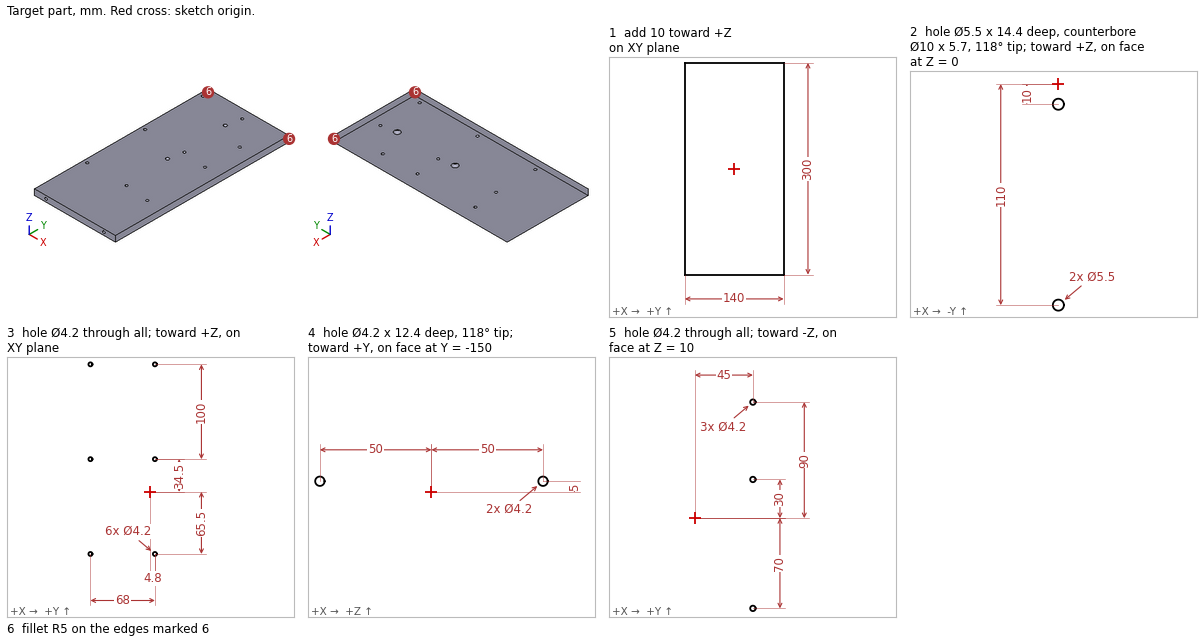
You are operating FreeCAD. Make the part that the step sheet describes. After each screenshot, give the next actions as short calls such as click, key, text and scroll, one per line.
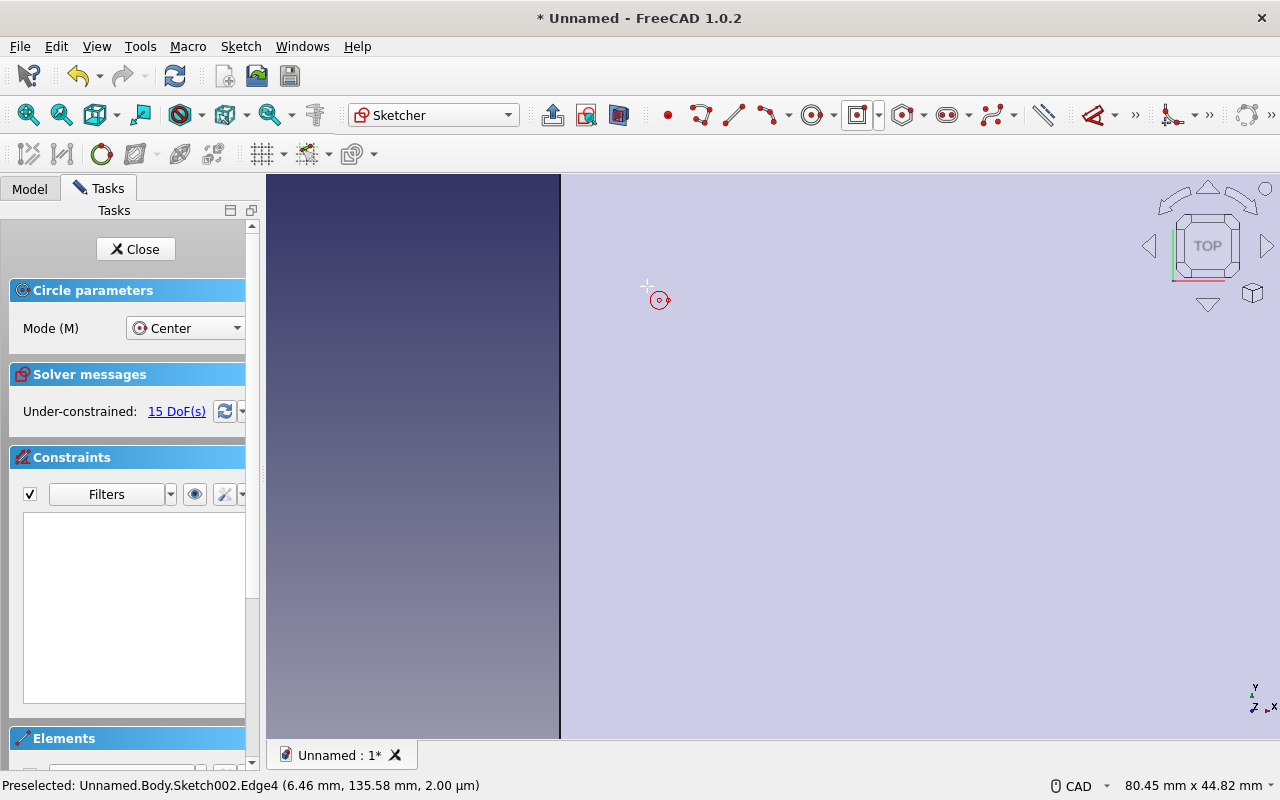
scroll(647, 286, down, 10)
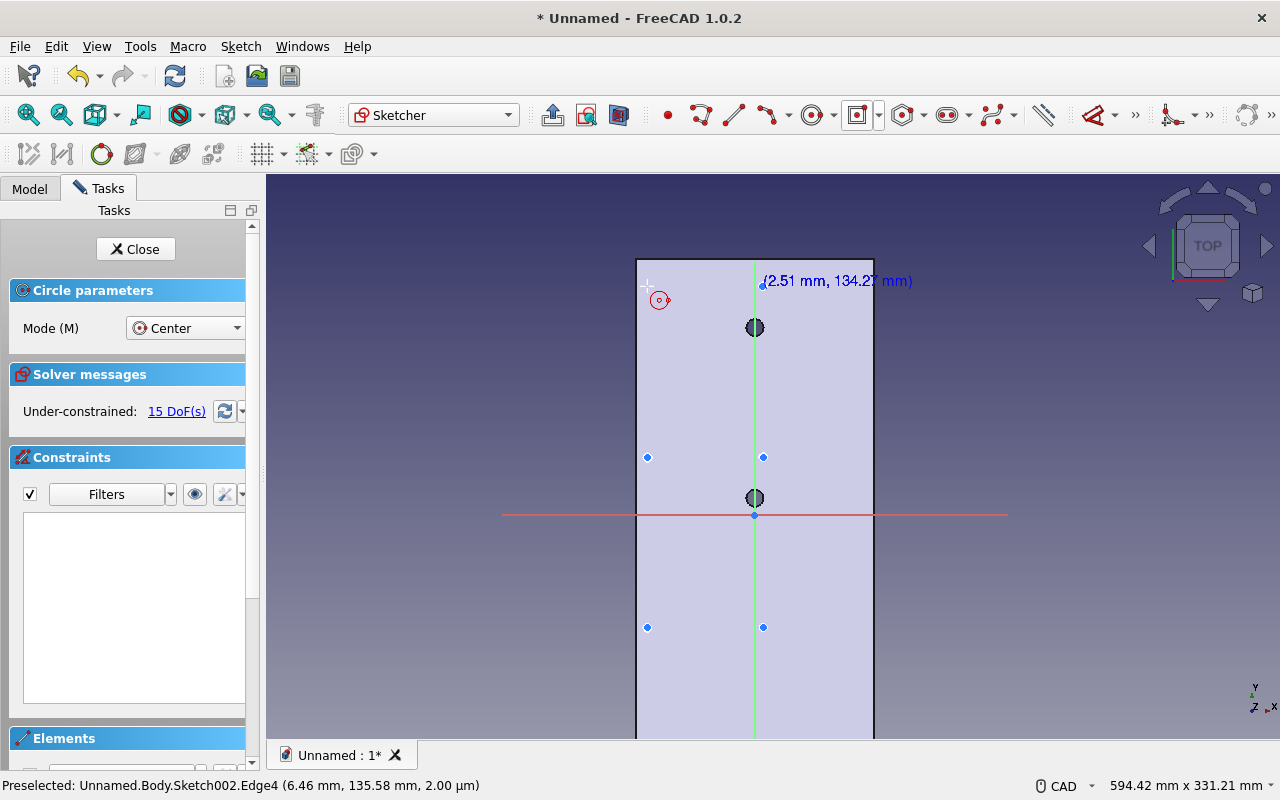
click(647, 286)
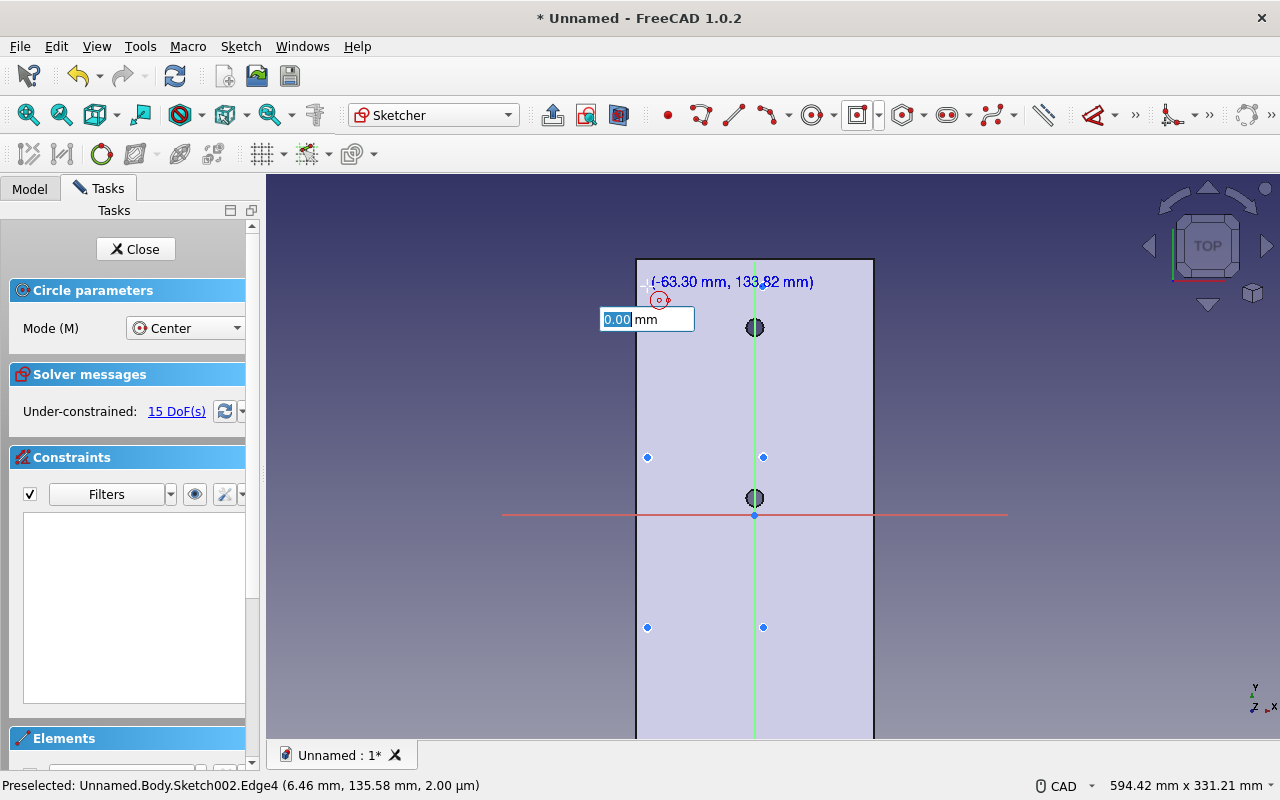
scroll(650, 283, up, 8)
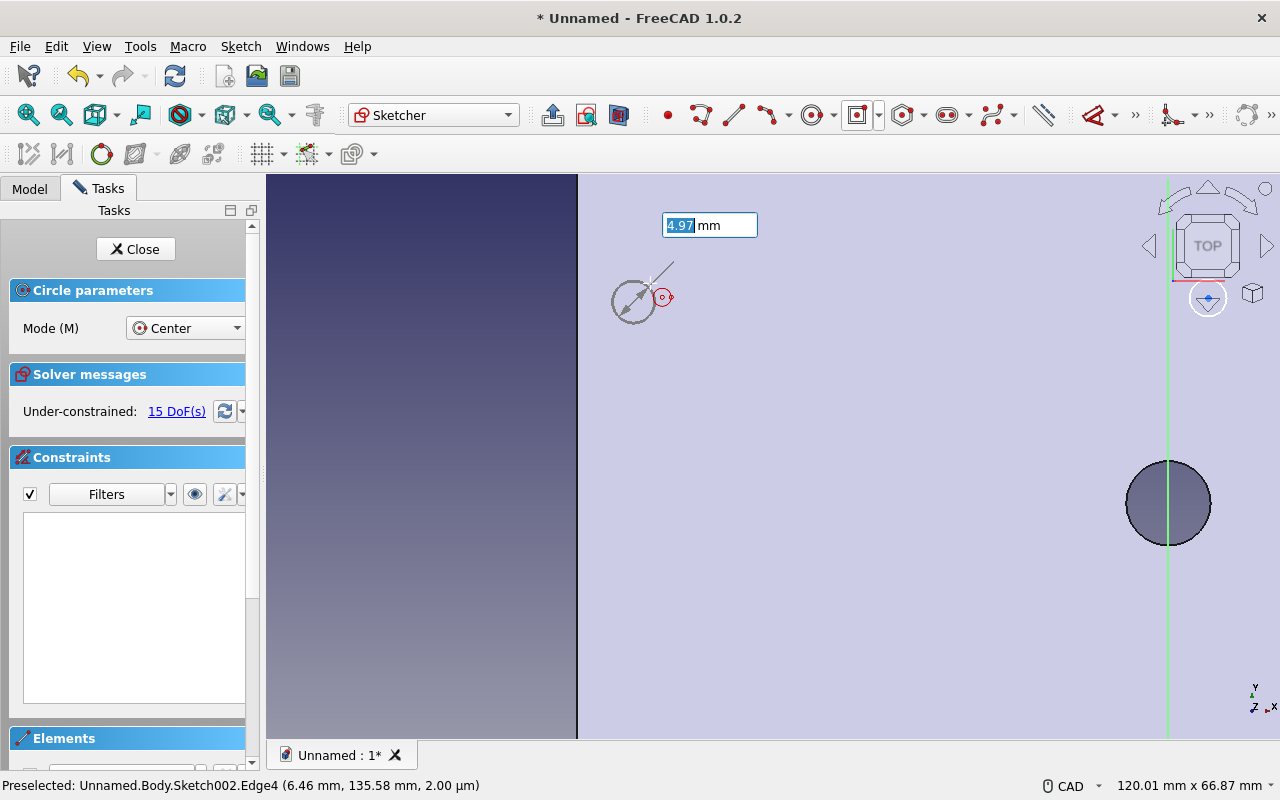
click(647, 284)
key(Escape)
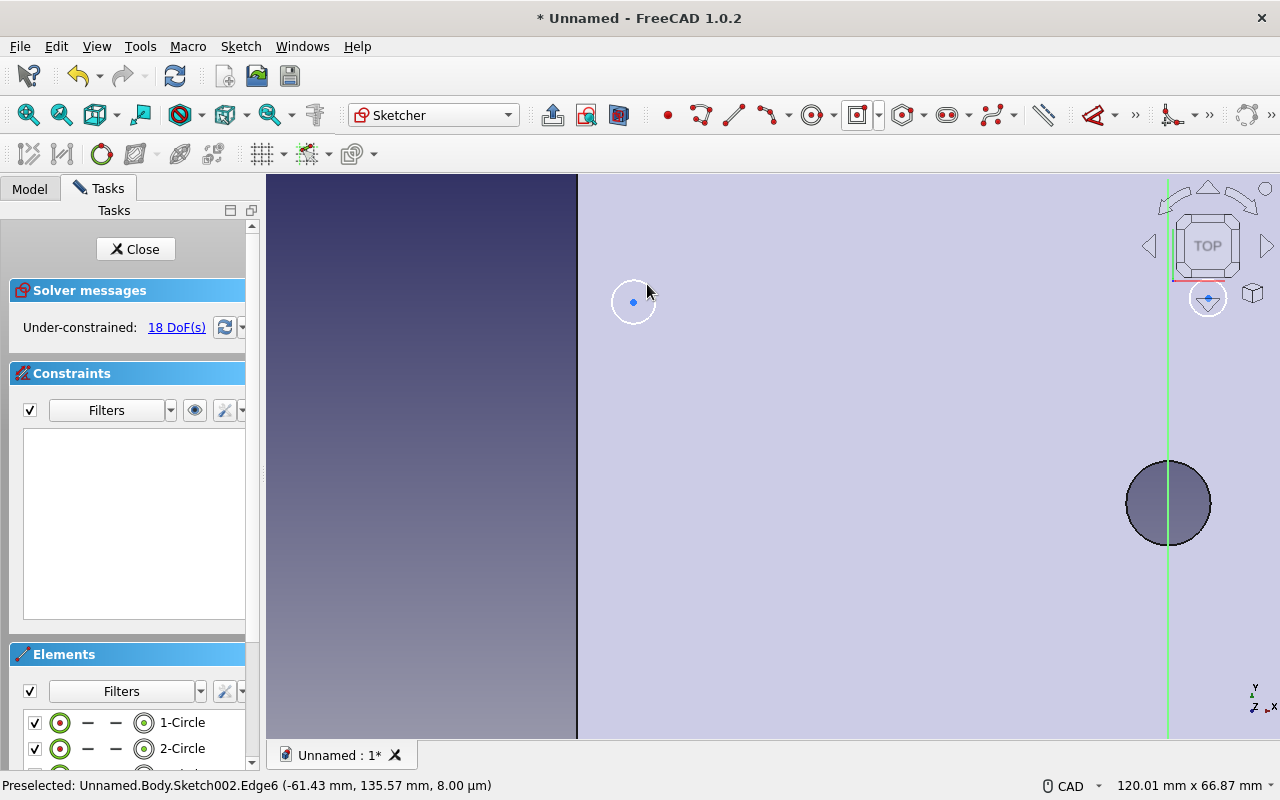
scroll(650, 283, down, 8)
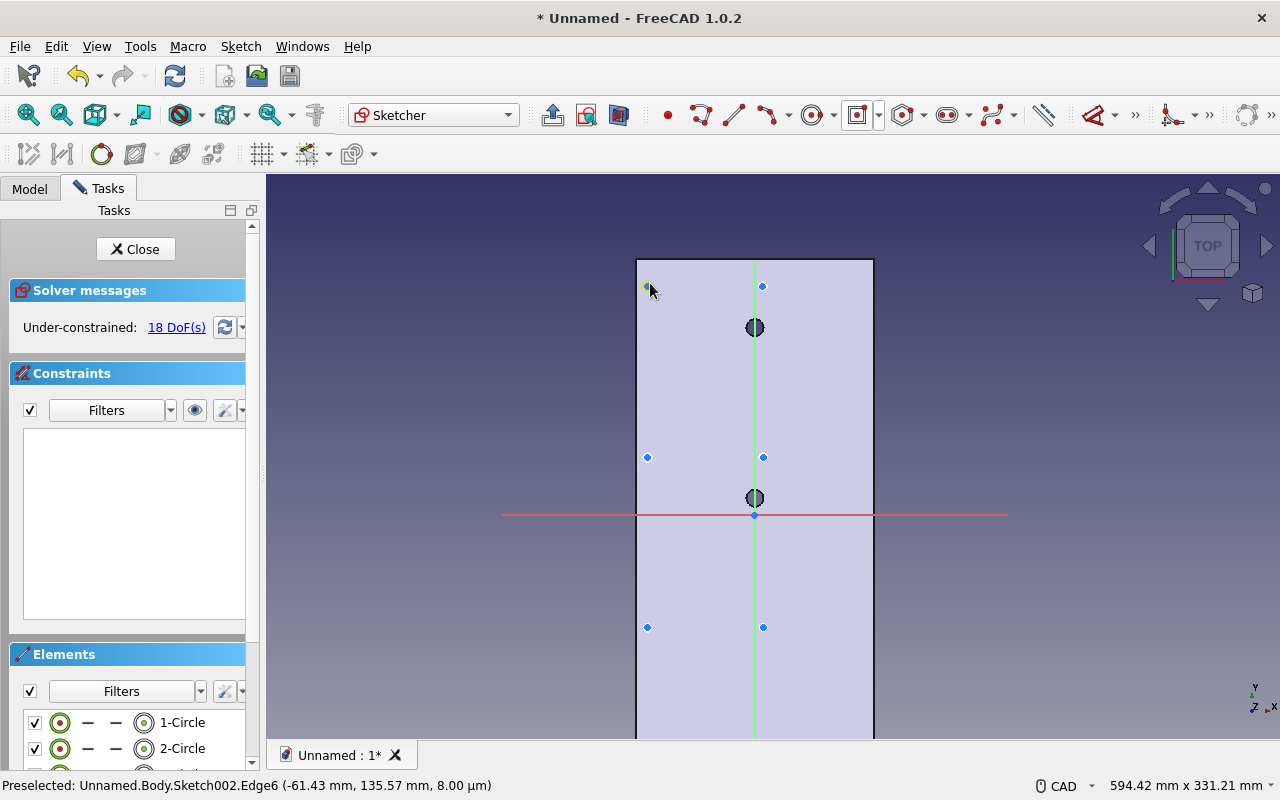
scroll(766, 625, up, 7)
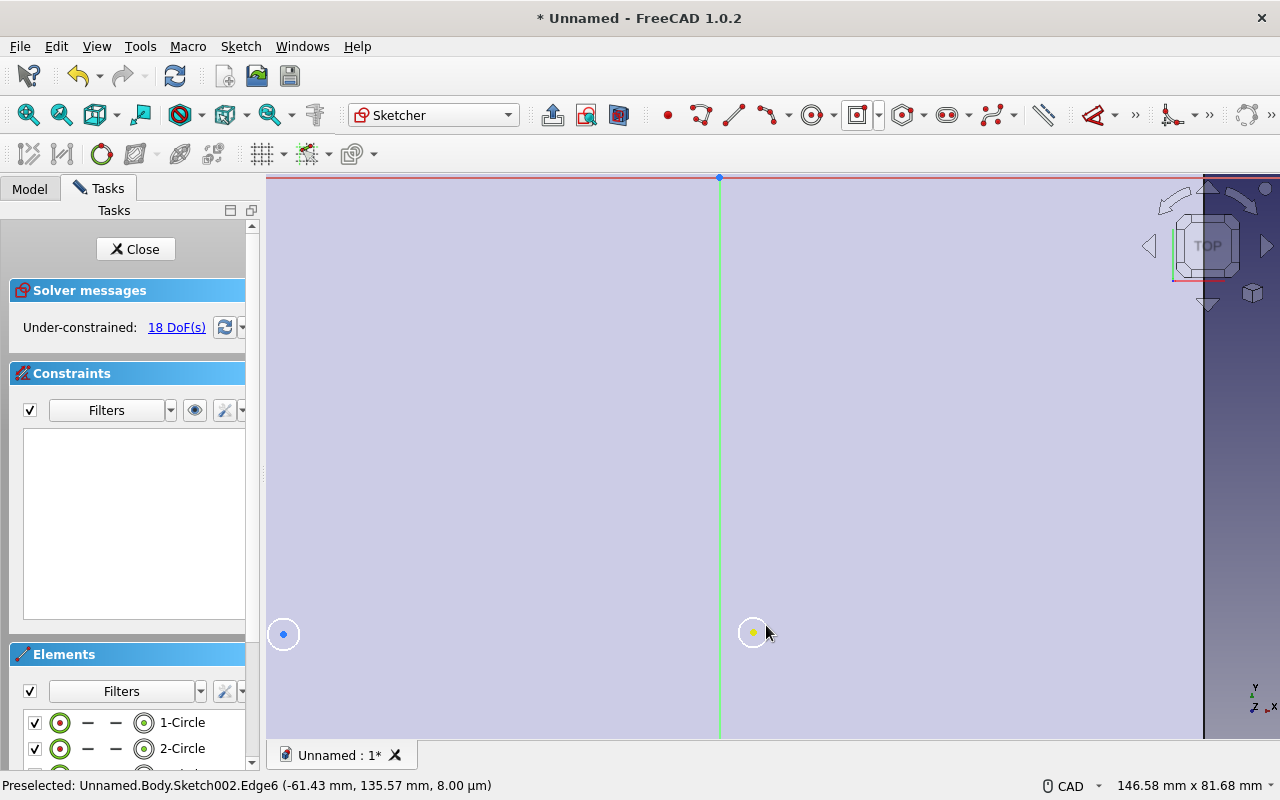
click(764, 622)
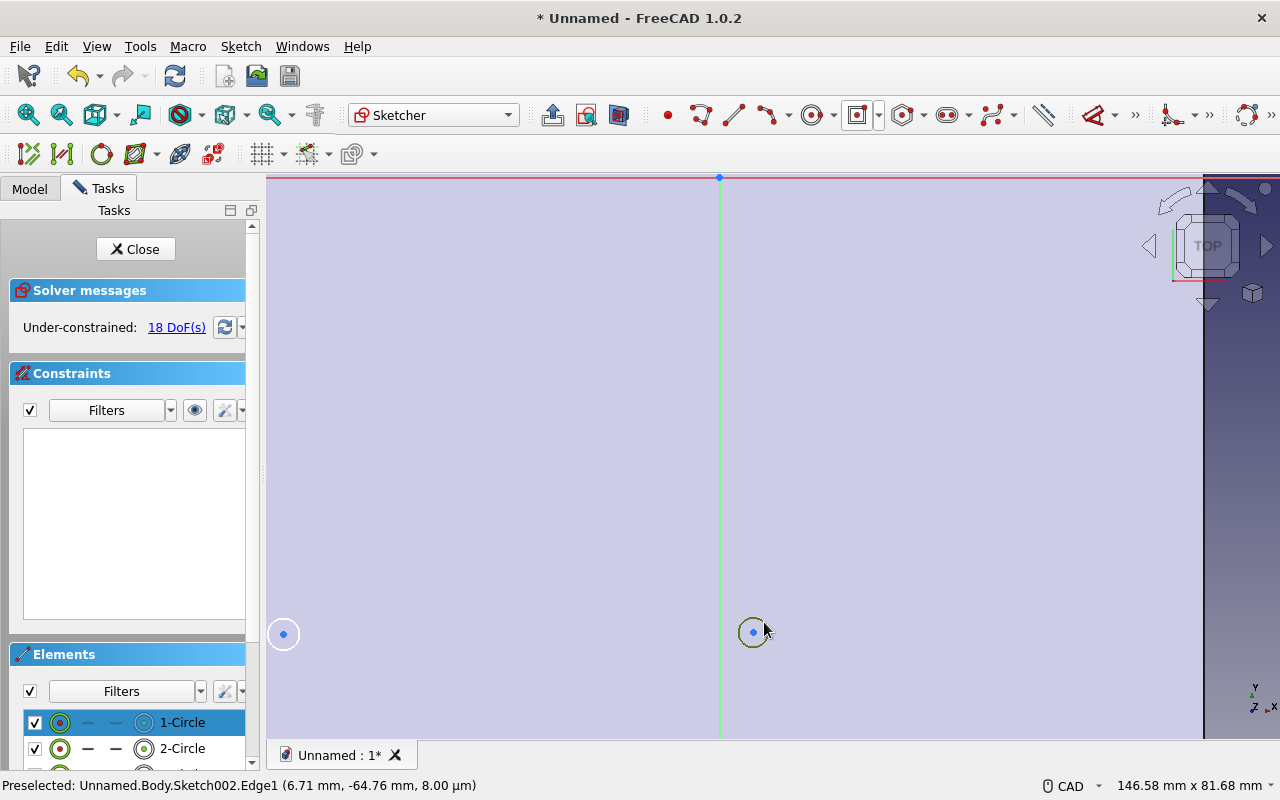
click(295, 623)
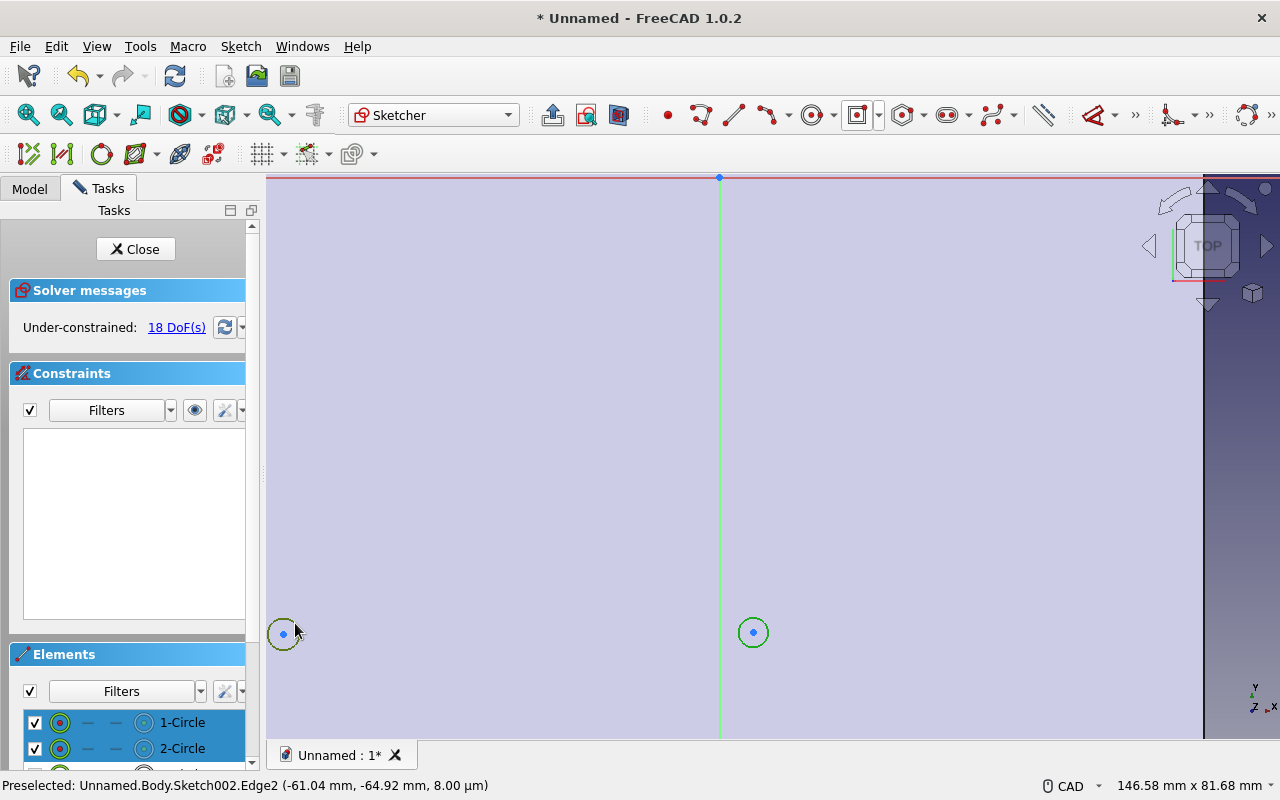
scroll(766, 626, down, 7)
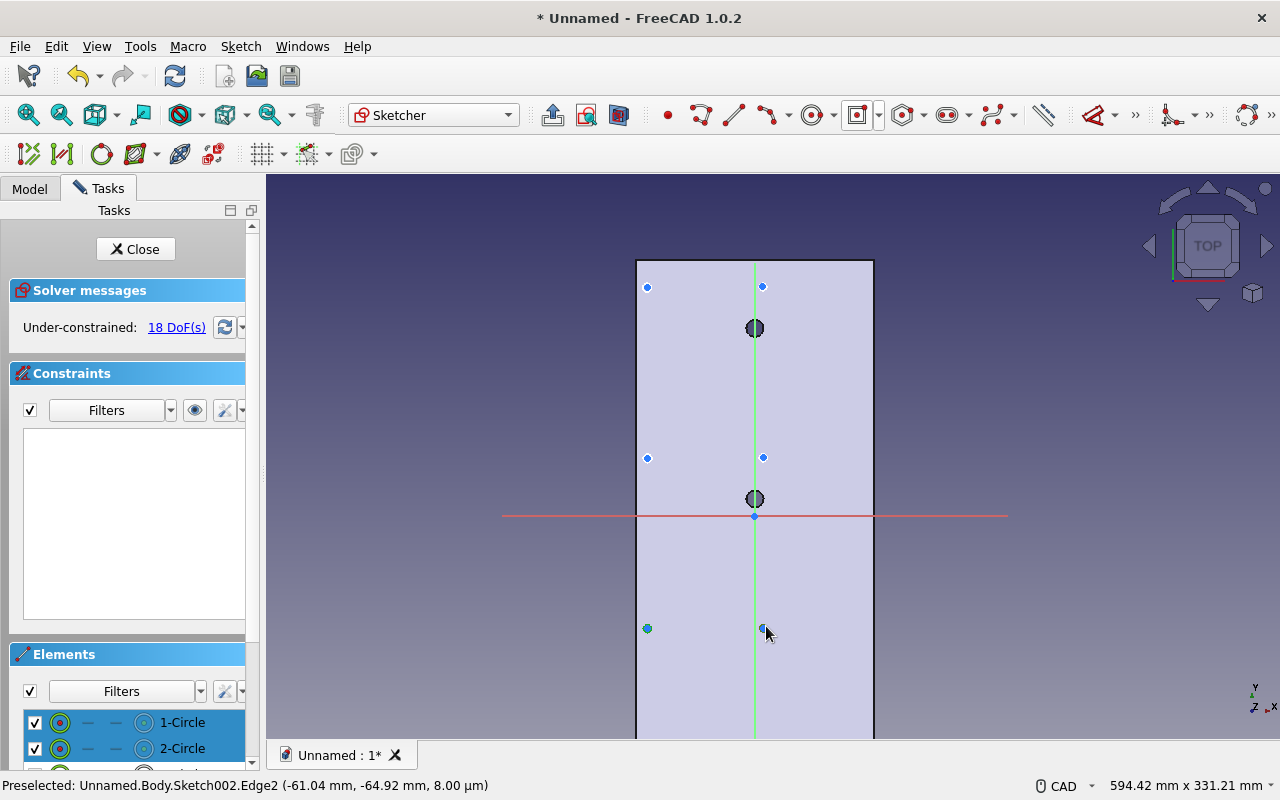
scroll(766, 455, up, 7)